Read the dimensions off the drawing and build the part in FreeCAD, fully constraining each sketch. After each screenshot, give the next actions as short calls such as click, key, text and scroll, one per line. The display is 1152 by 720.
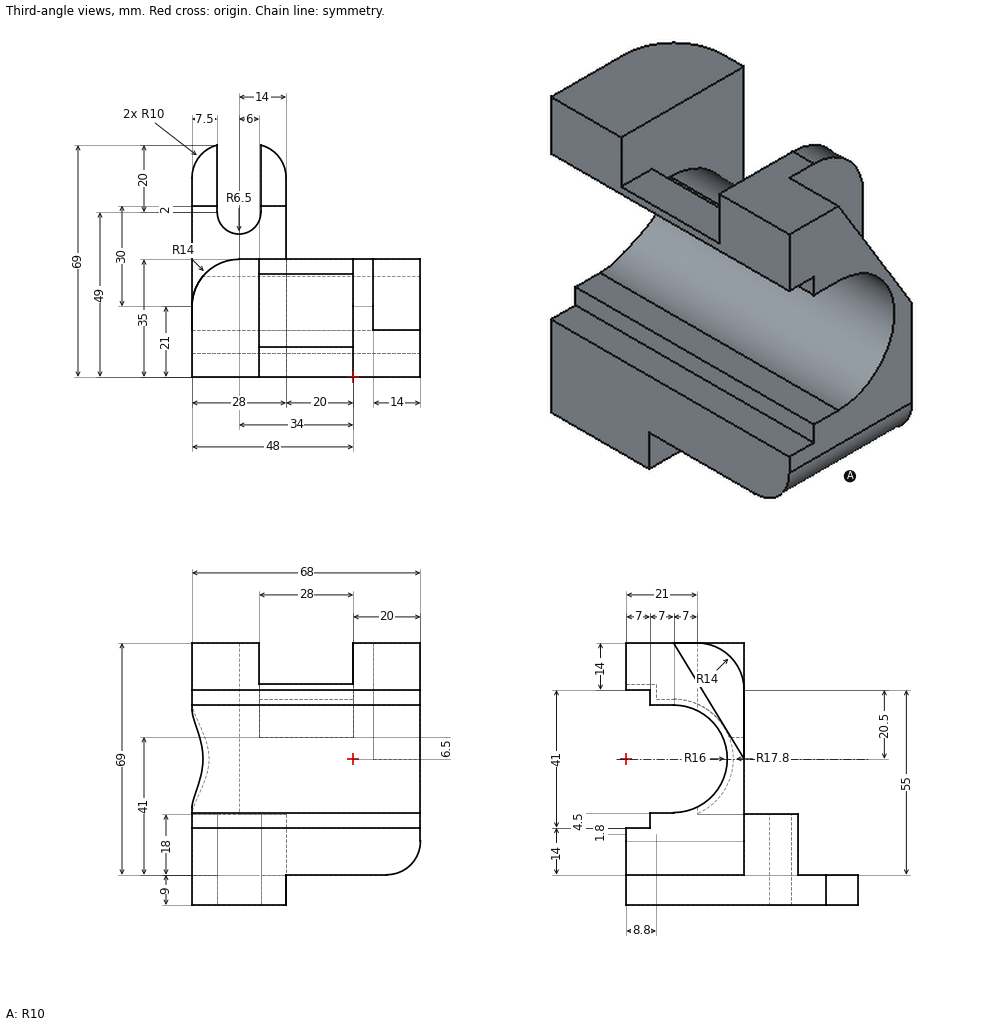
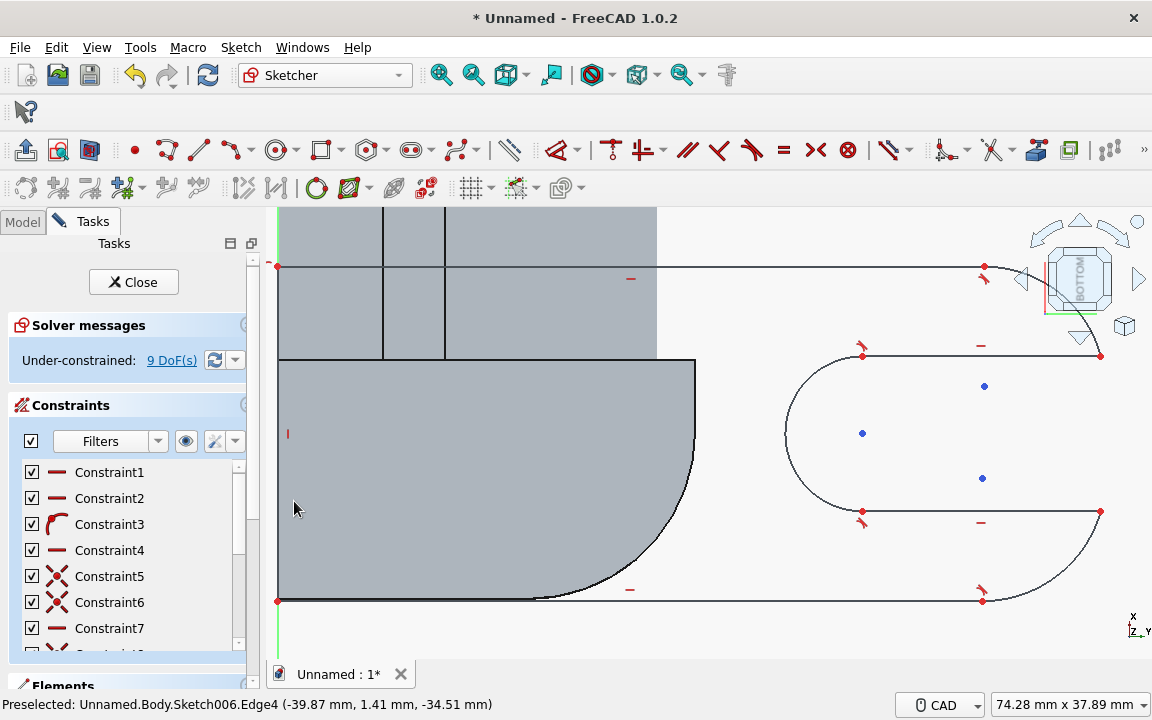
scroll(601, 531, down, 4)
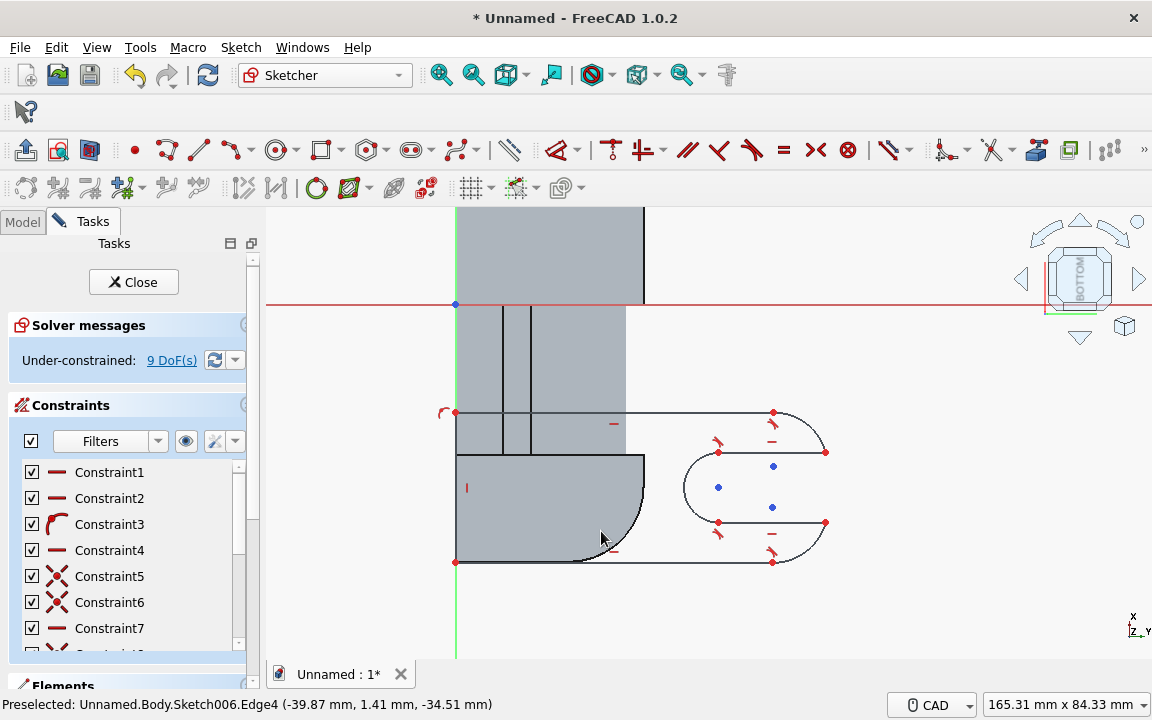
click(817, 434)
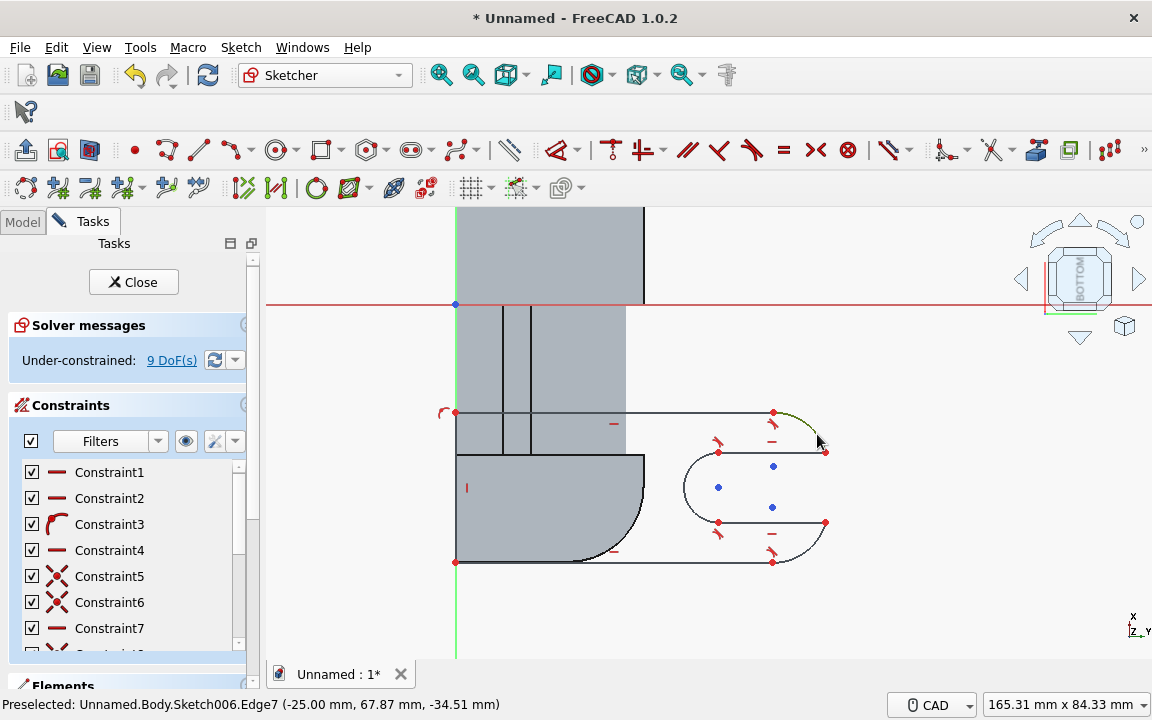
click(794, 559)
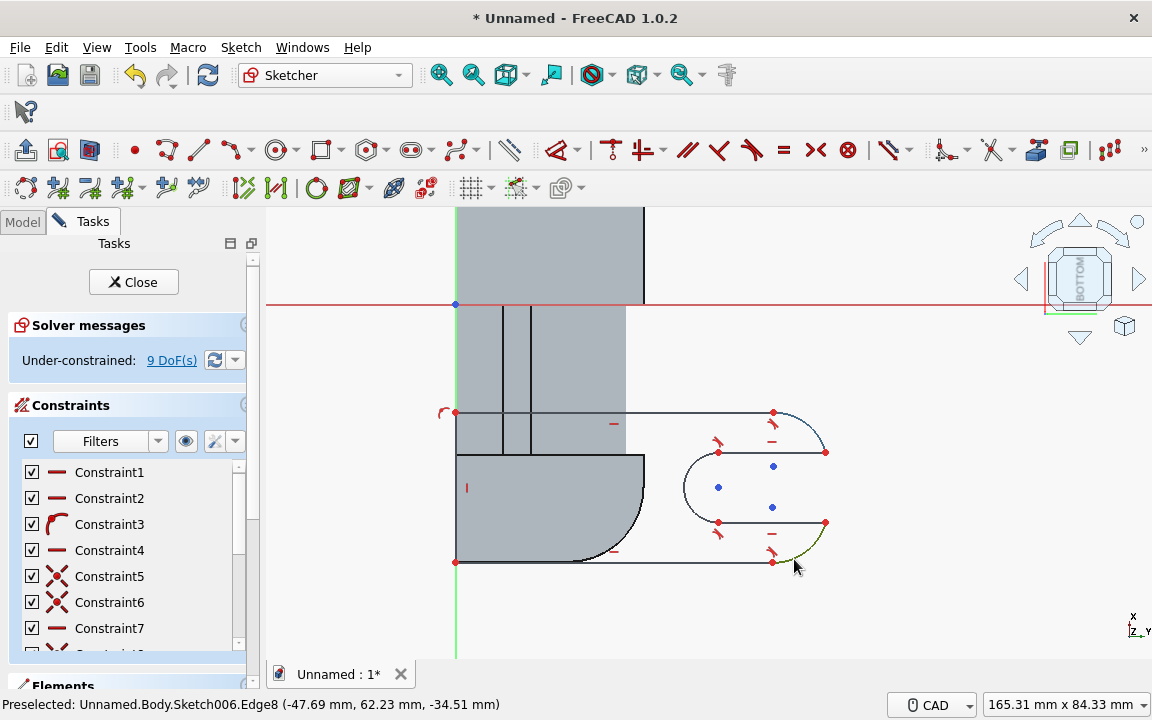
key(e)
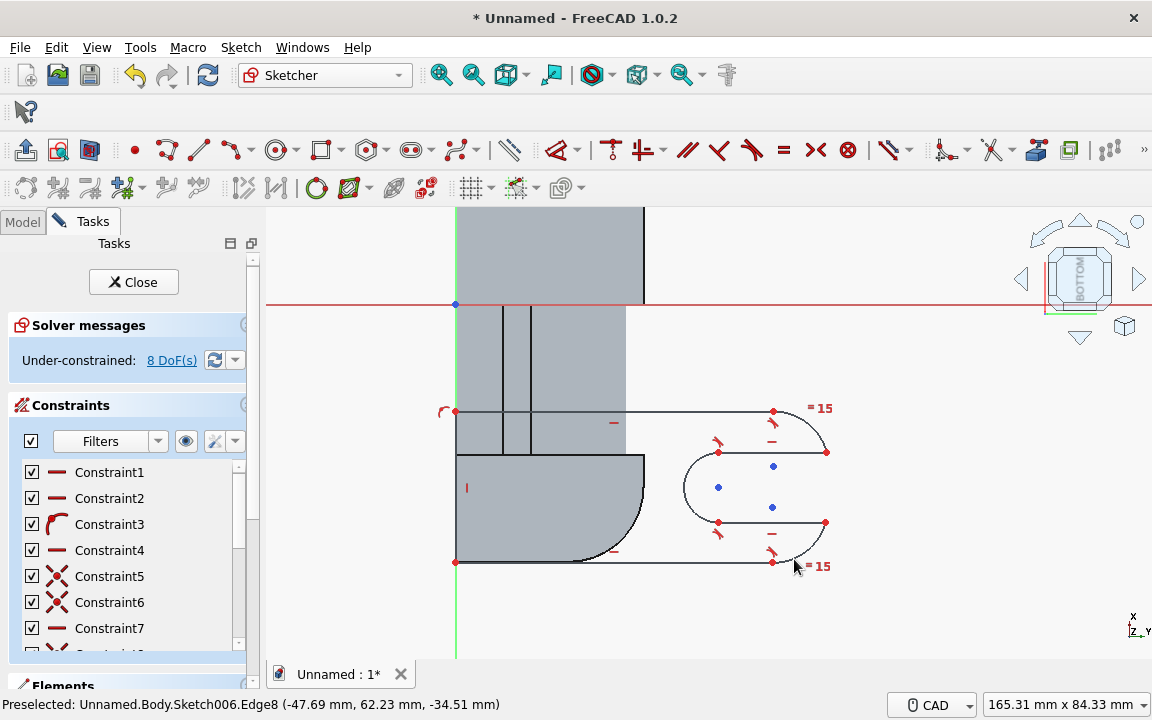
click(556, 150)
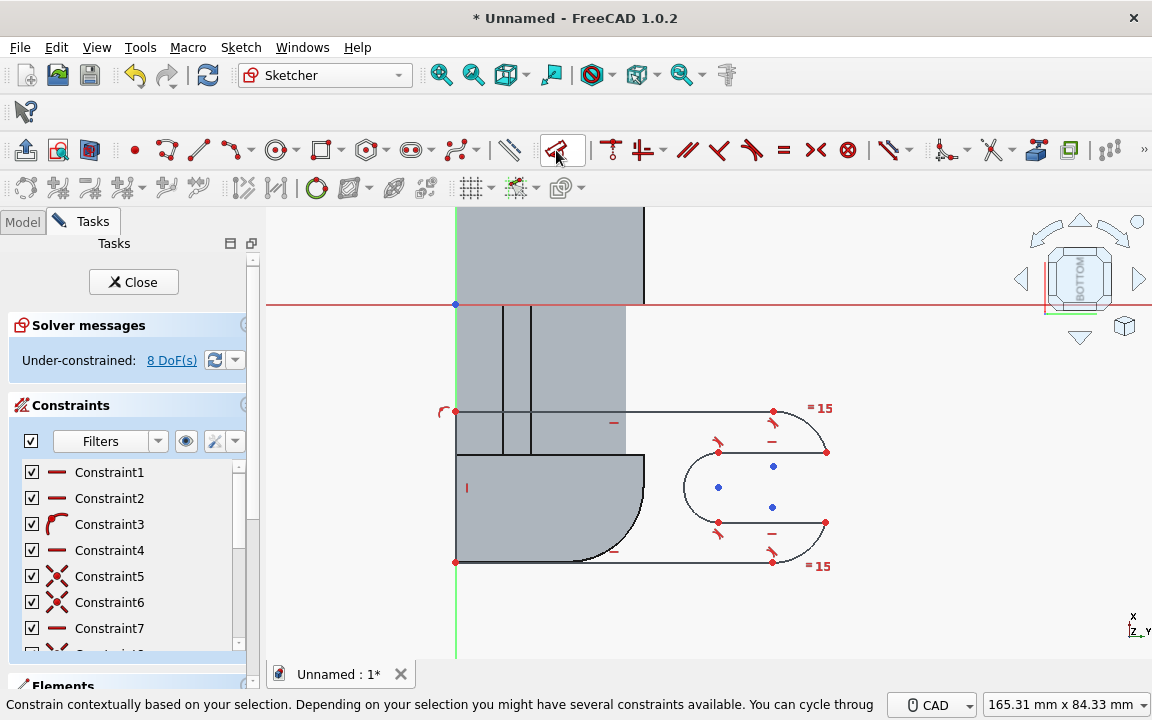
click(691, 467)
click(665, 448)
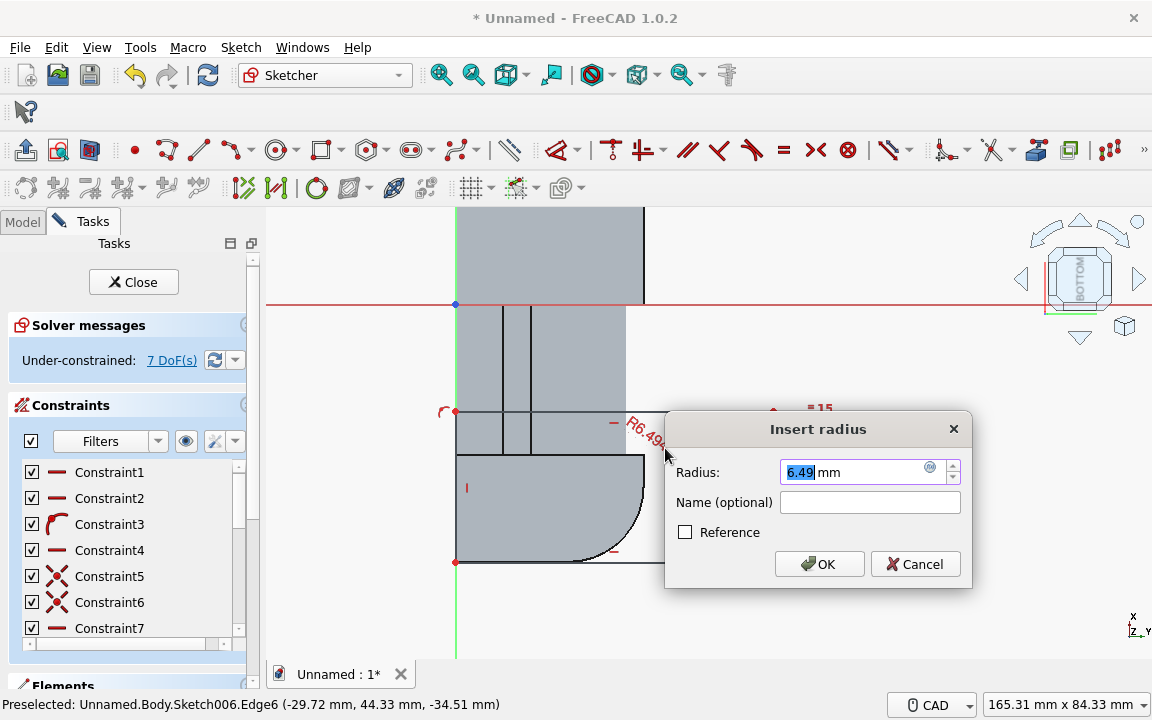
text(6.5)
key(Return)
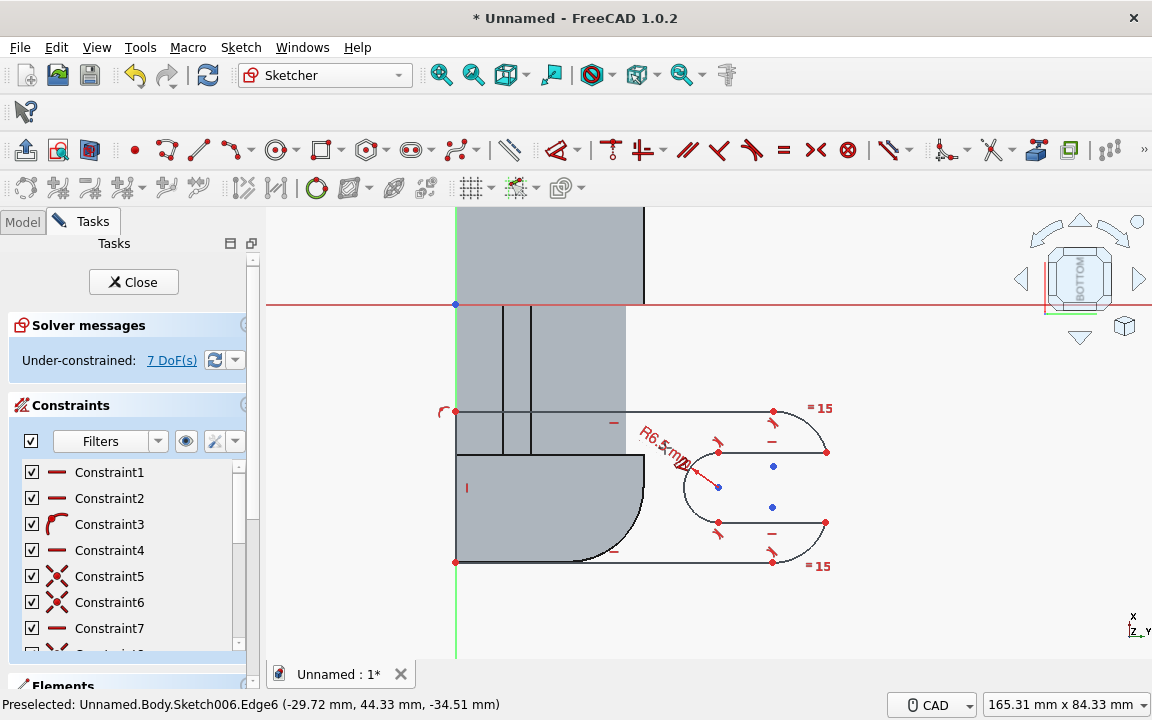
click(817, 433)
click(842, 413)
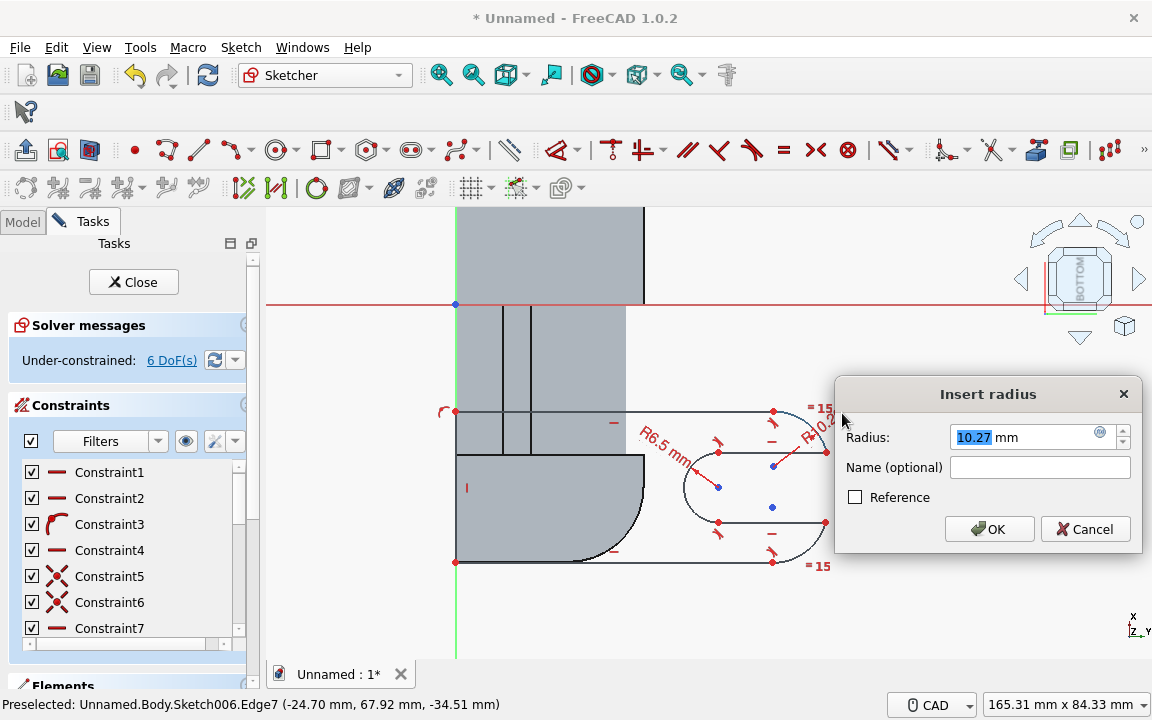
text(10)
key(Return)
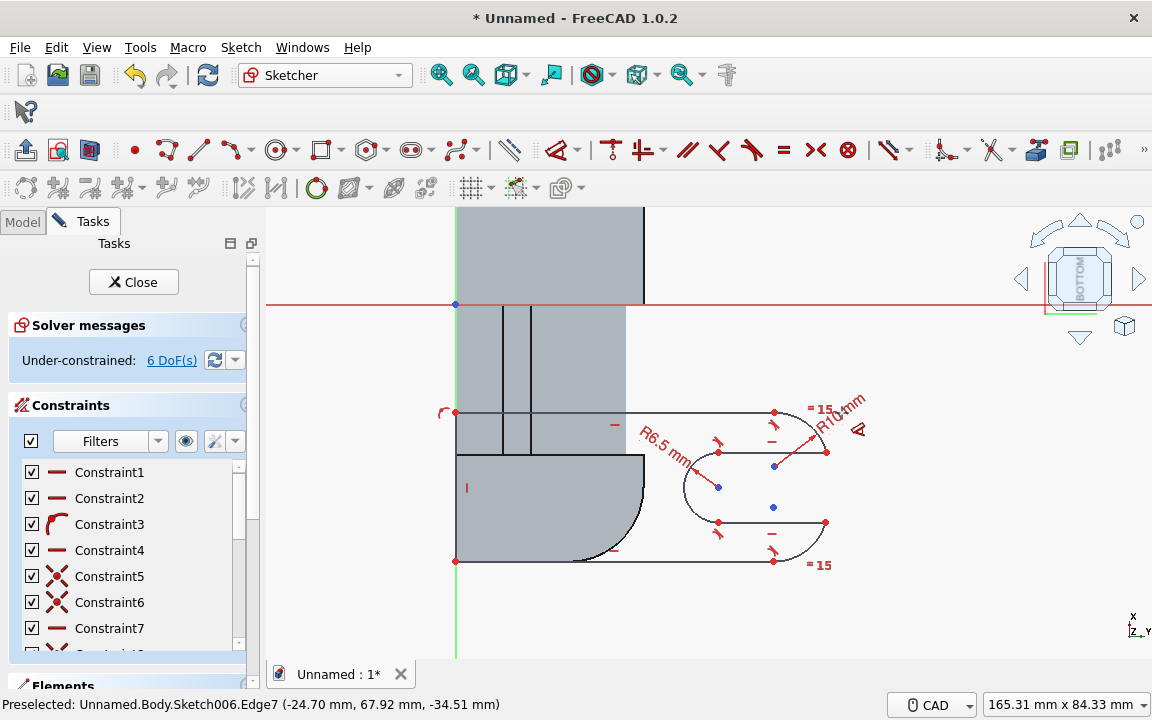
click(794, 523)
click(772, 489)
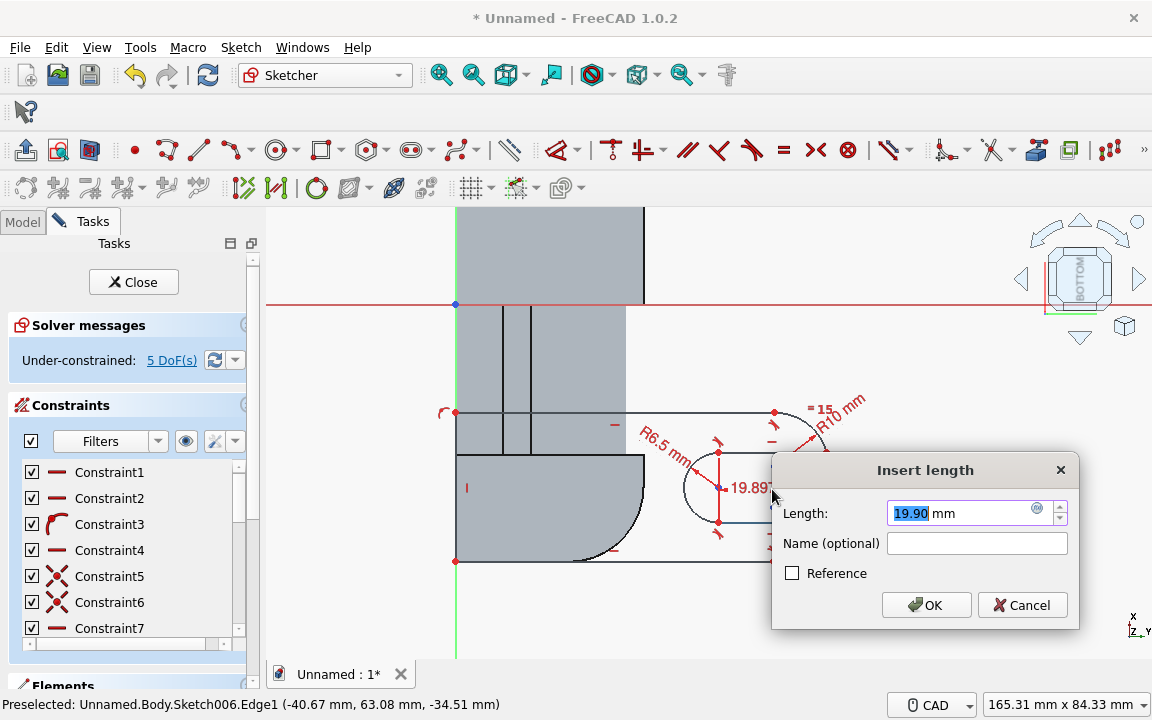
text(20)
key(Return)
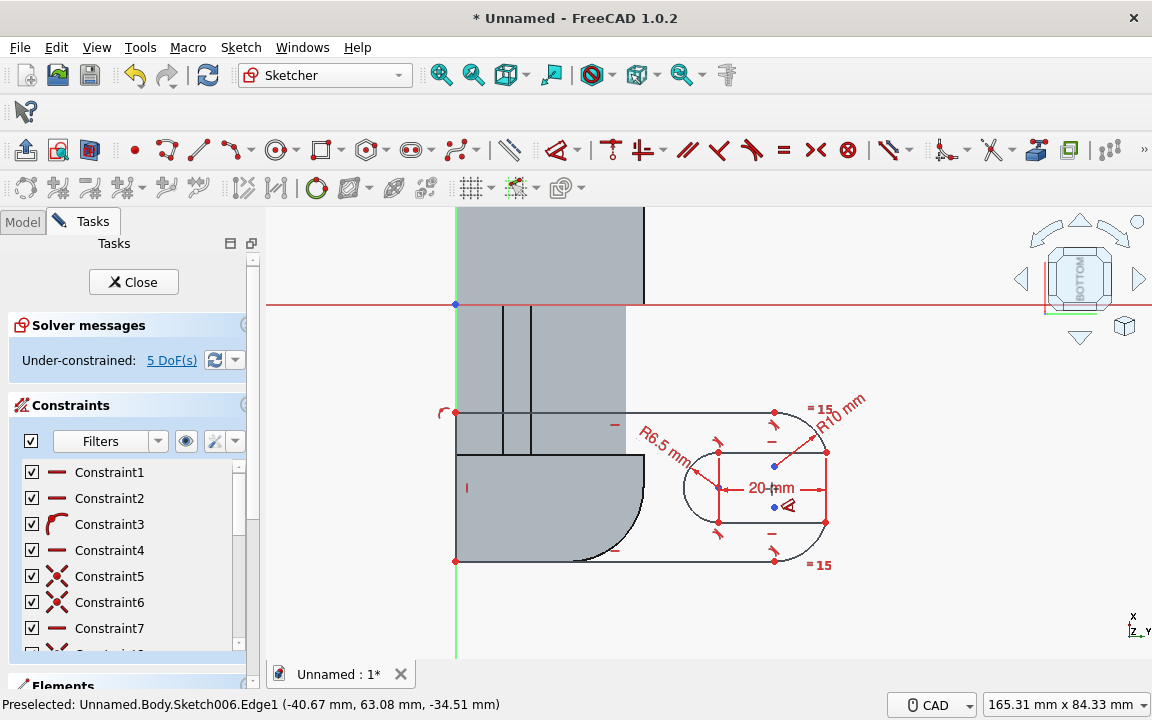
click(751, 453)
click(748, 395)